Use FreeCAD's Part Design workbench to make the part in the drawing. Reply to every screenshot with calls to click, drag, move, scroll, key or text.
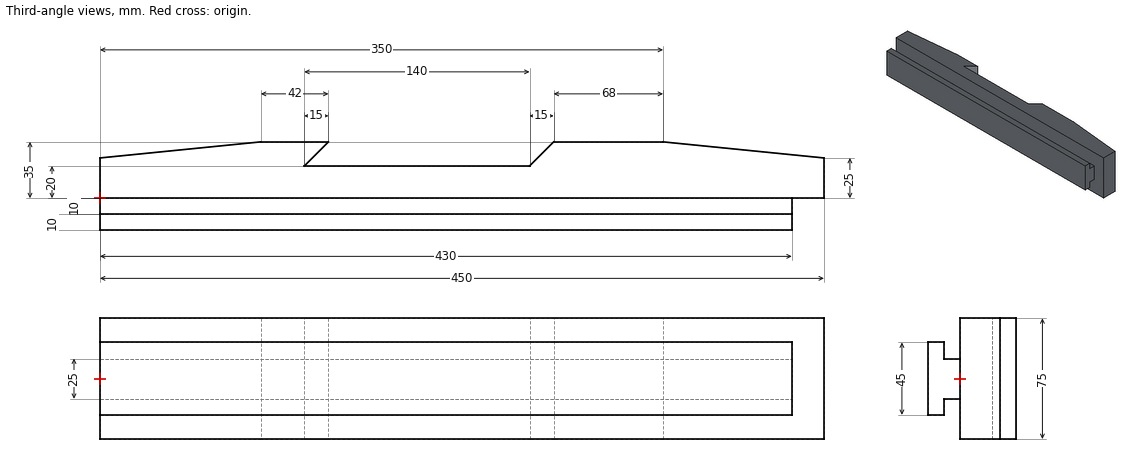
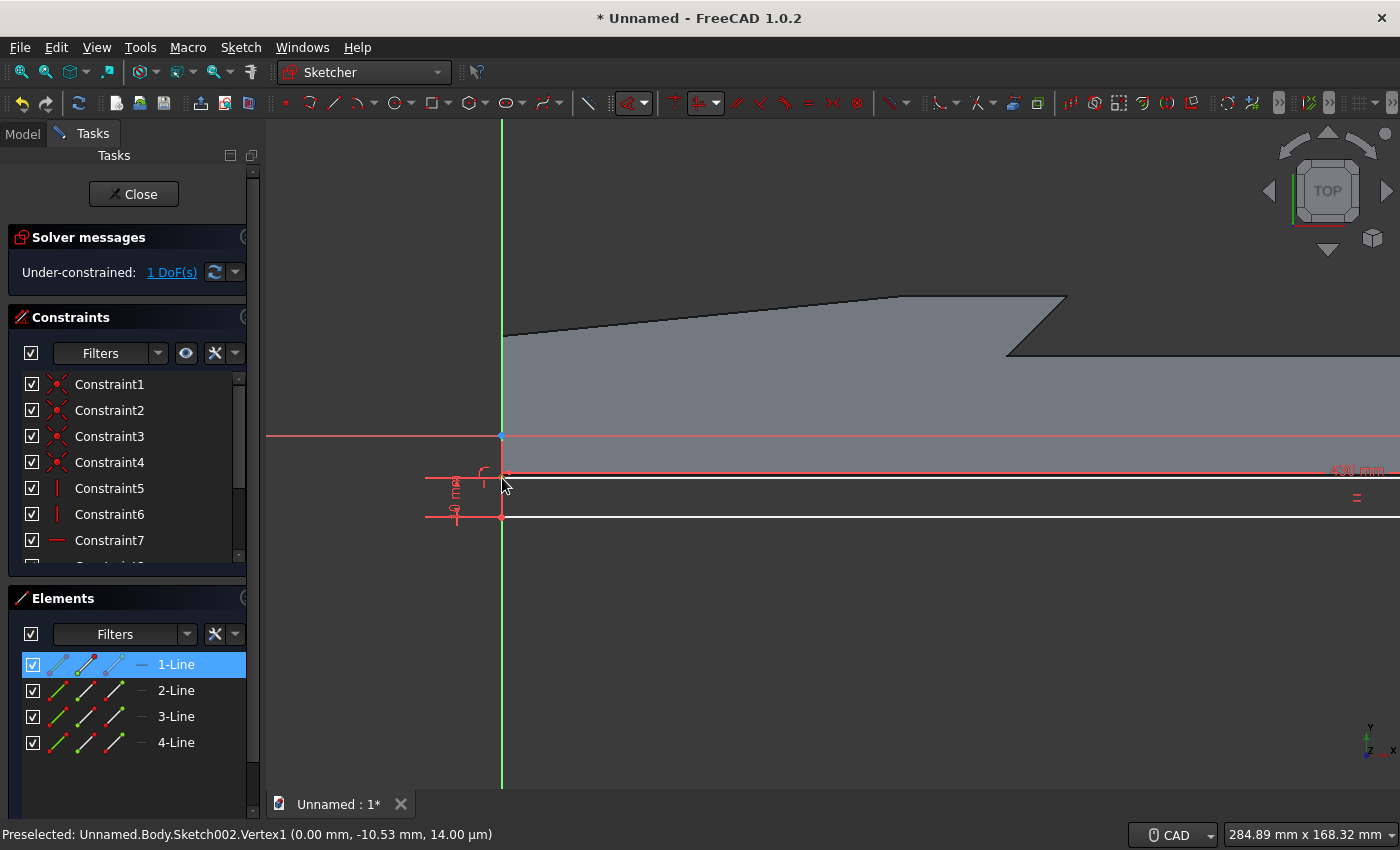
click(646, 104)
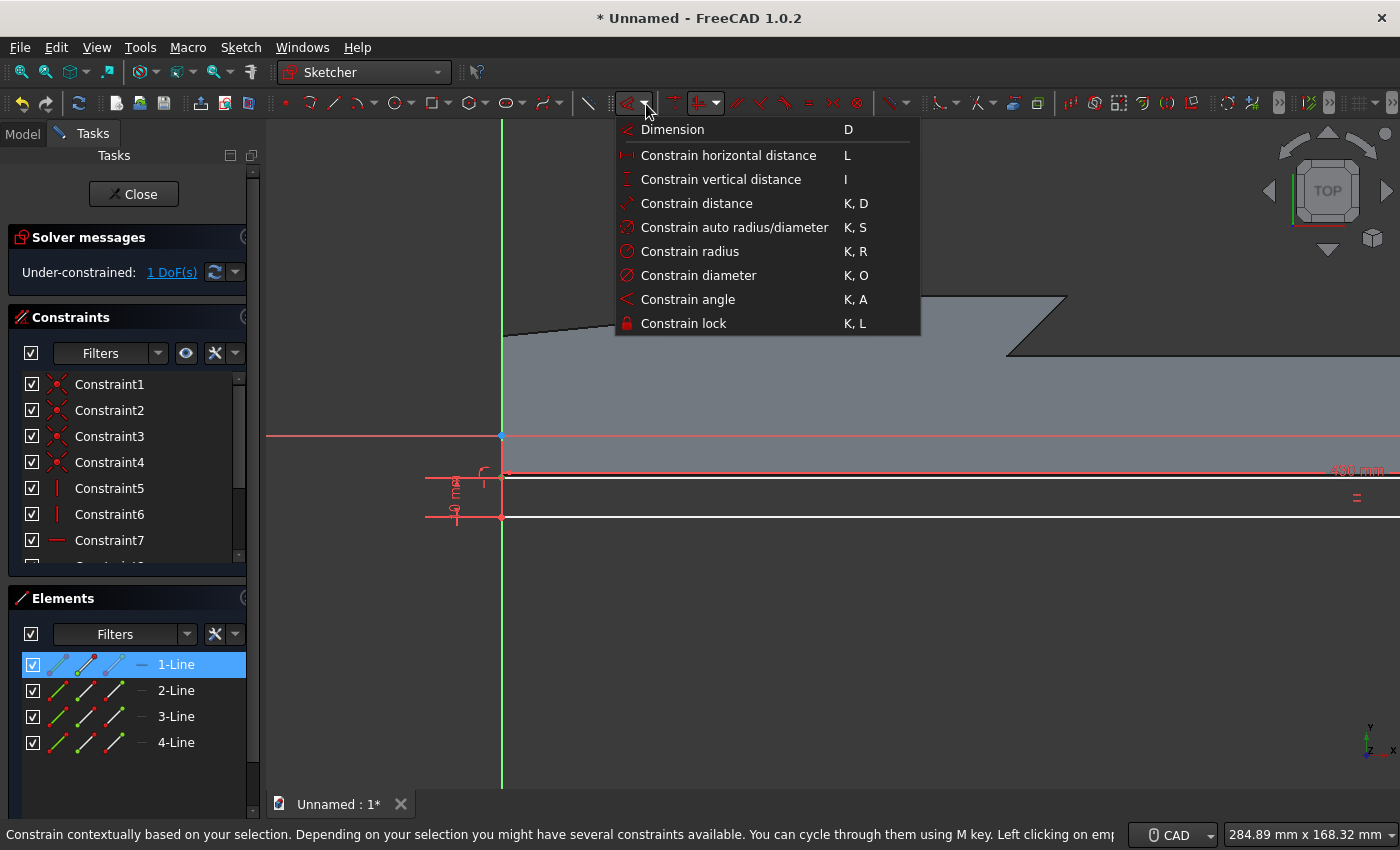
click(768, 179)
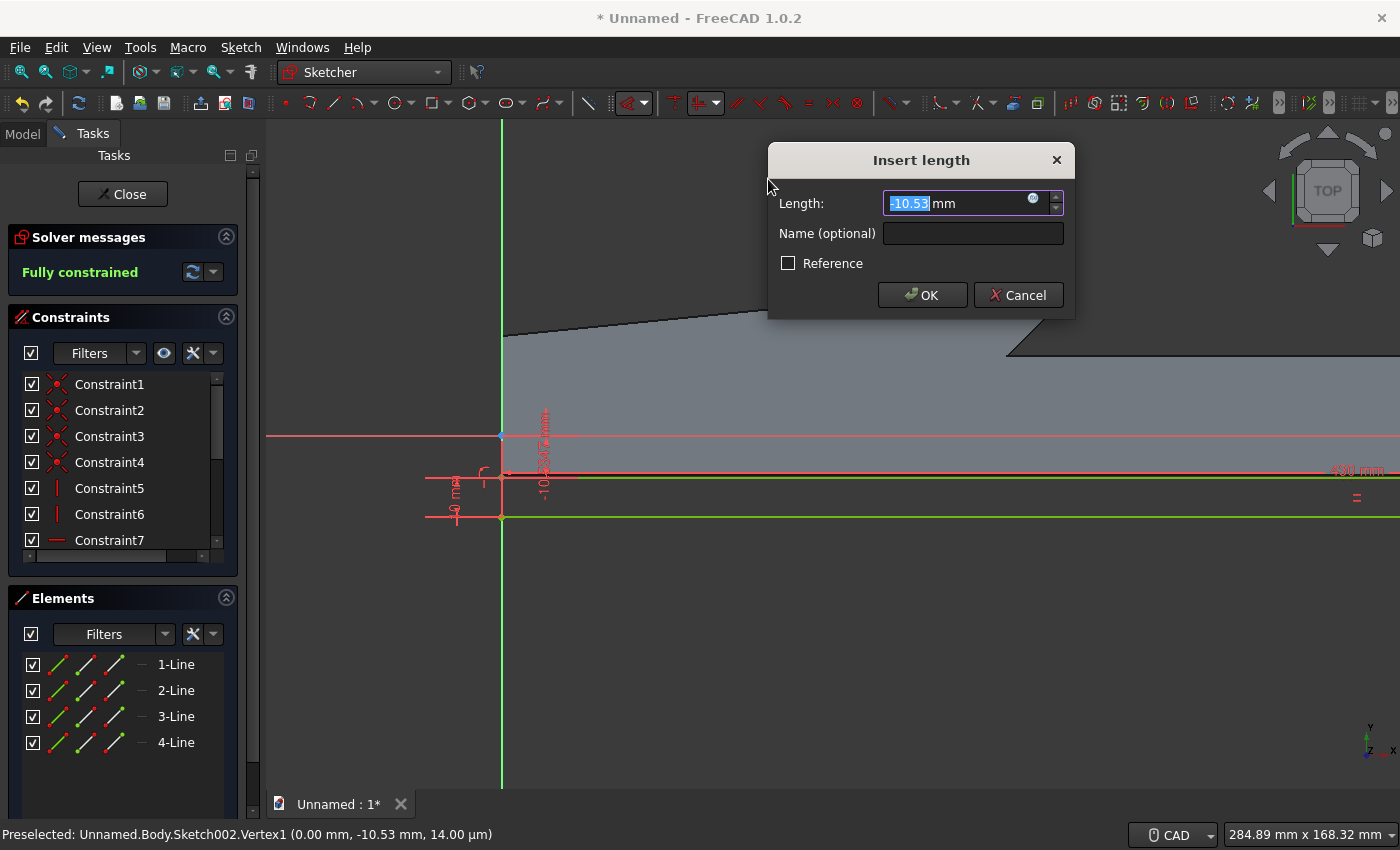
text(-10)
key(Return)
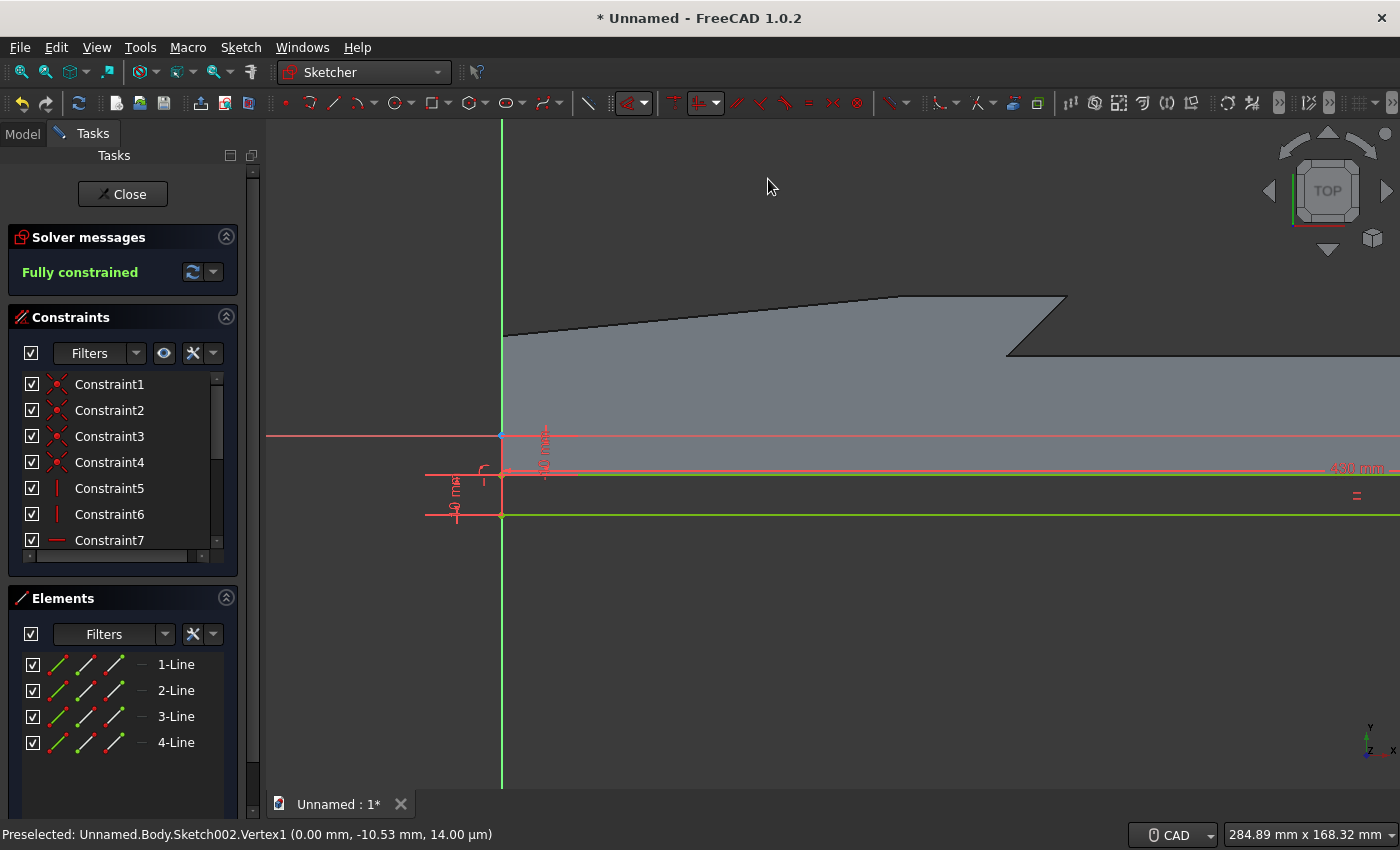
click(123, 194)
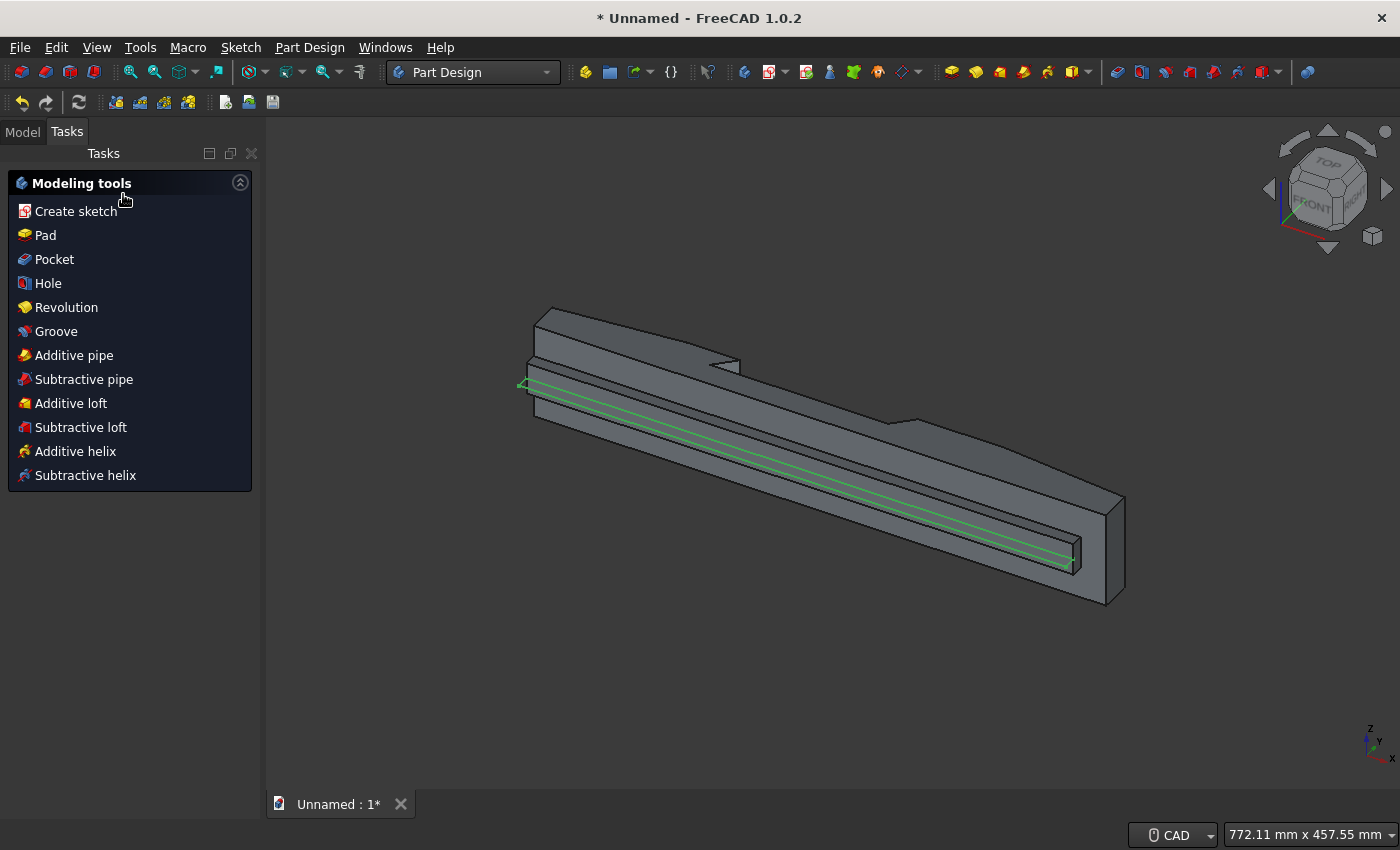
click(952, 72)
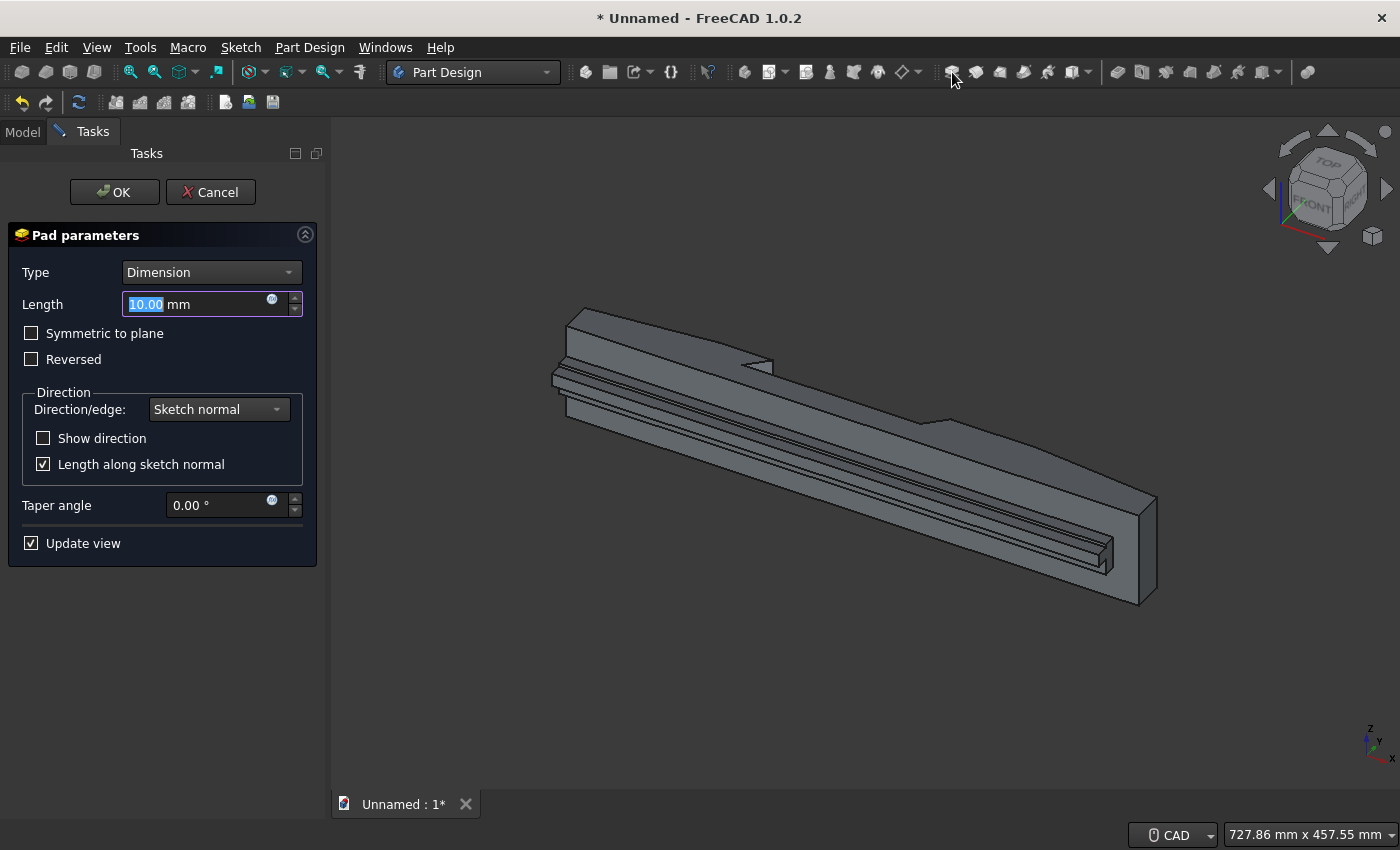
text(45)
key(Tab)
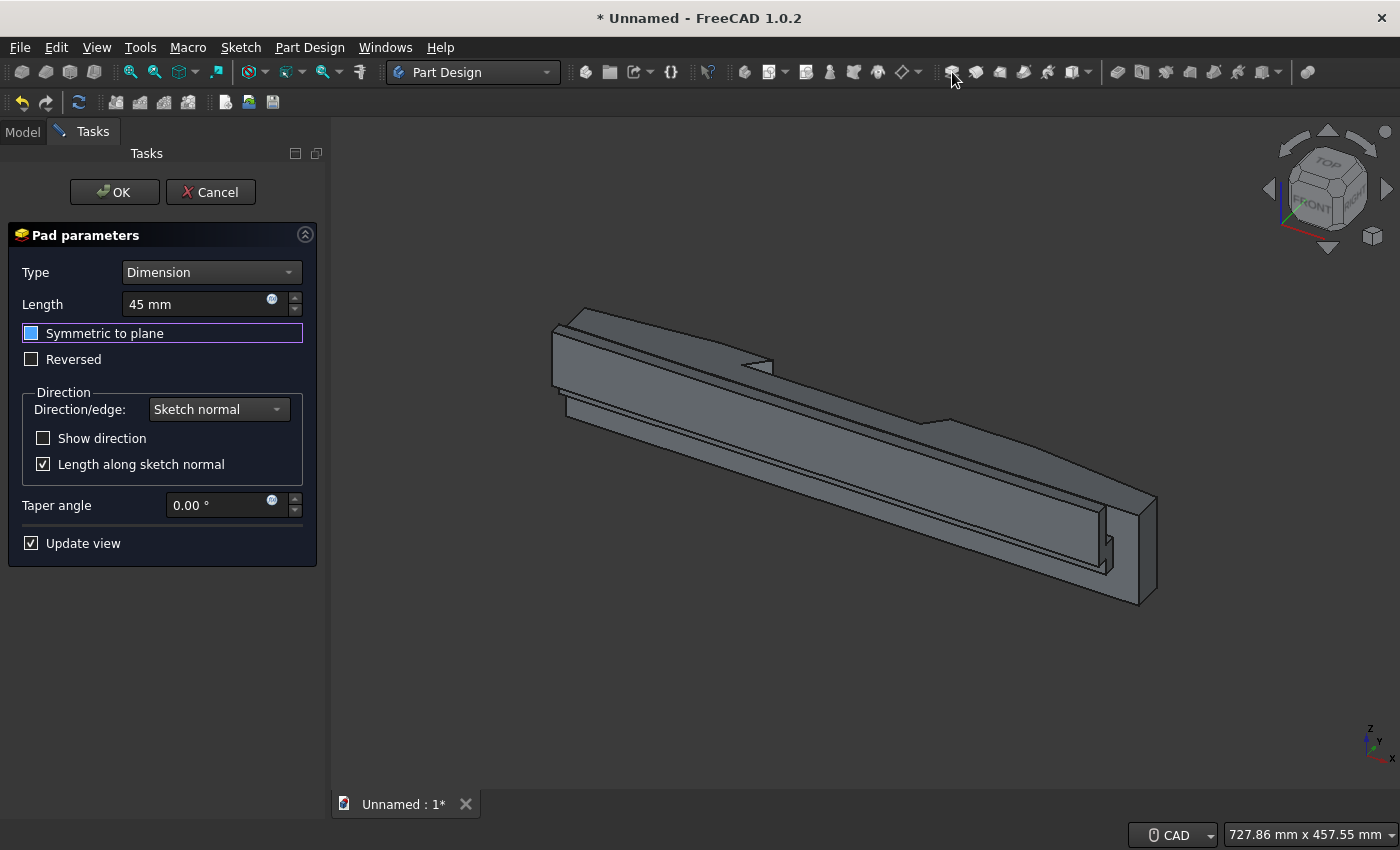
click(30, 333)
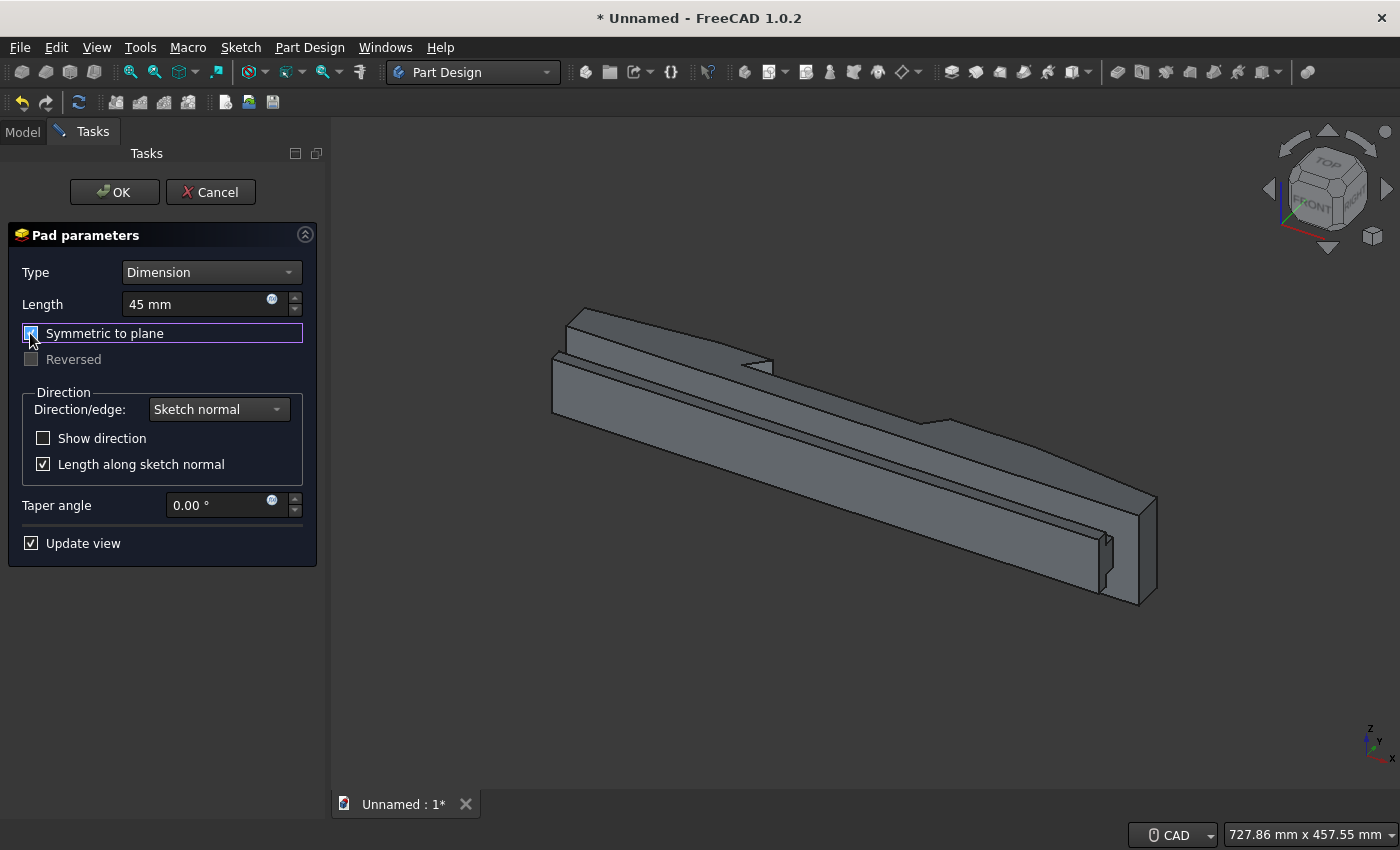
click(115, 192)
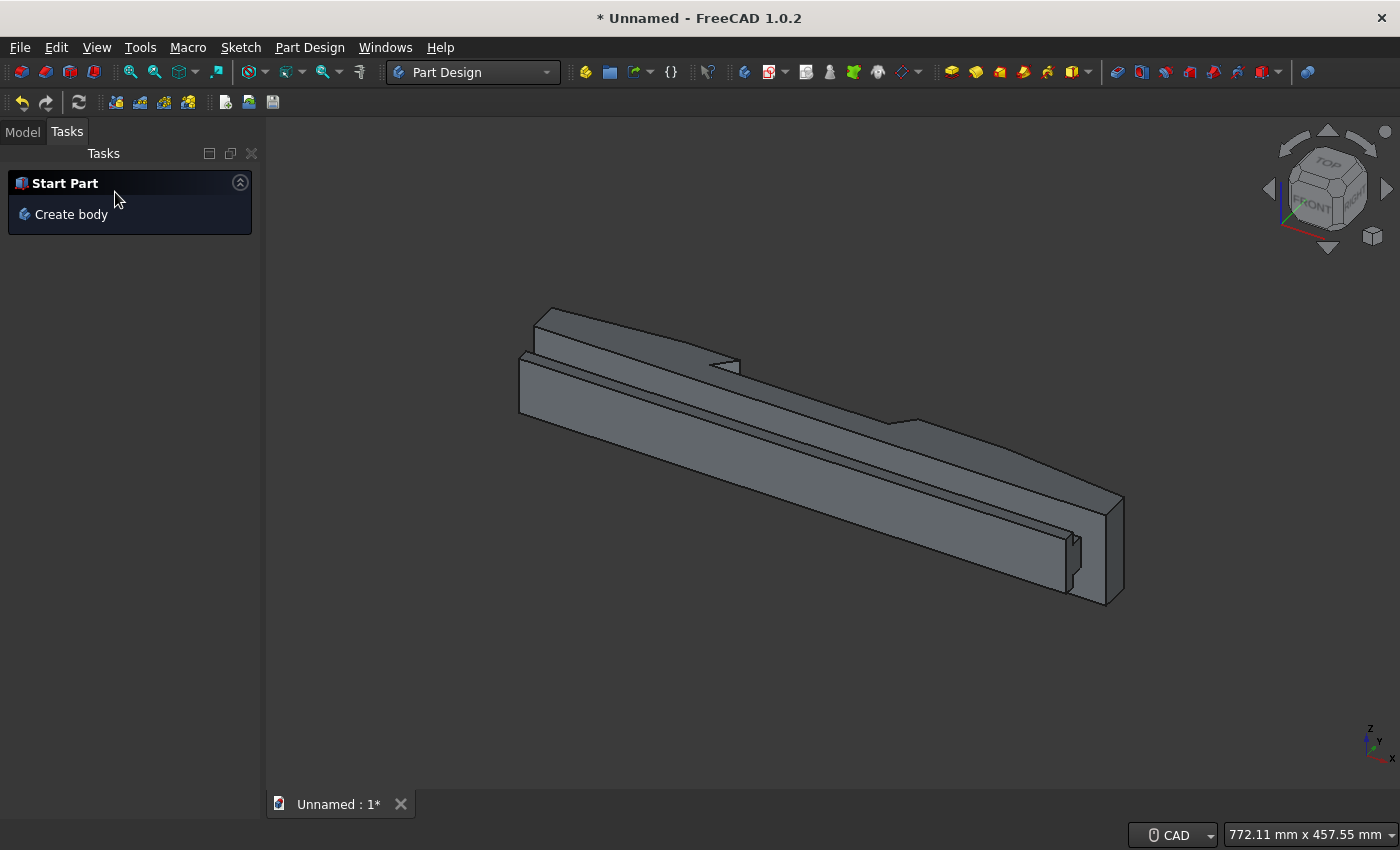
key(0)